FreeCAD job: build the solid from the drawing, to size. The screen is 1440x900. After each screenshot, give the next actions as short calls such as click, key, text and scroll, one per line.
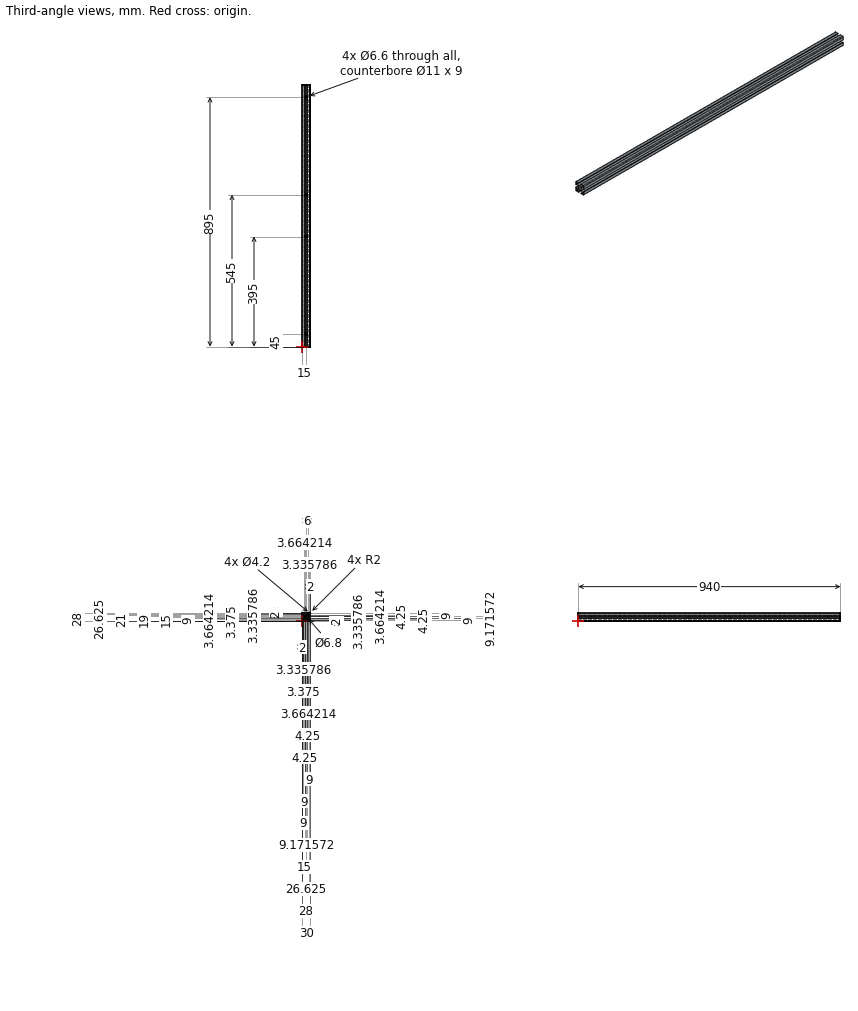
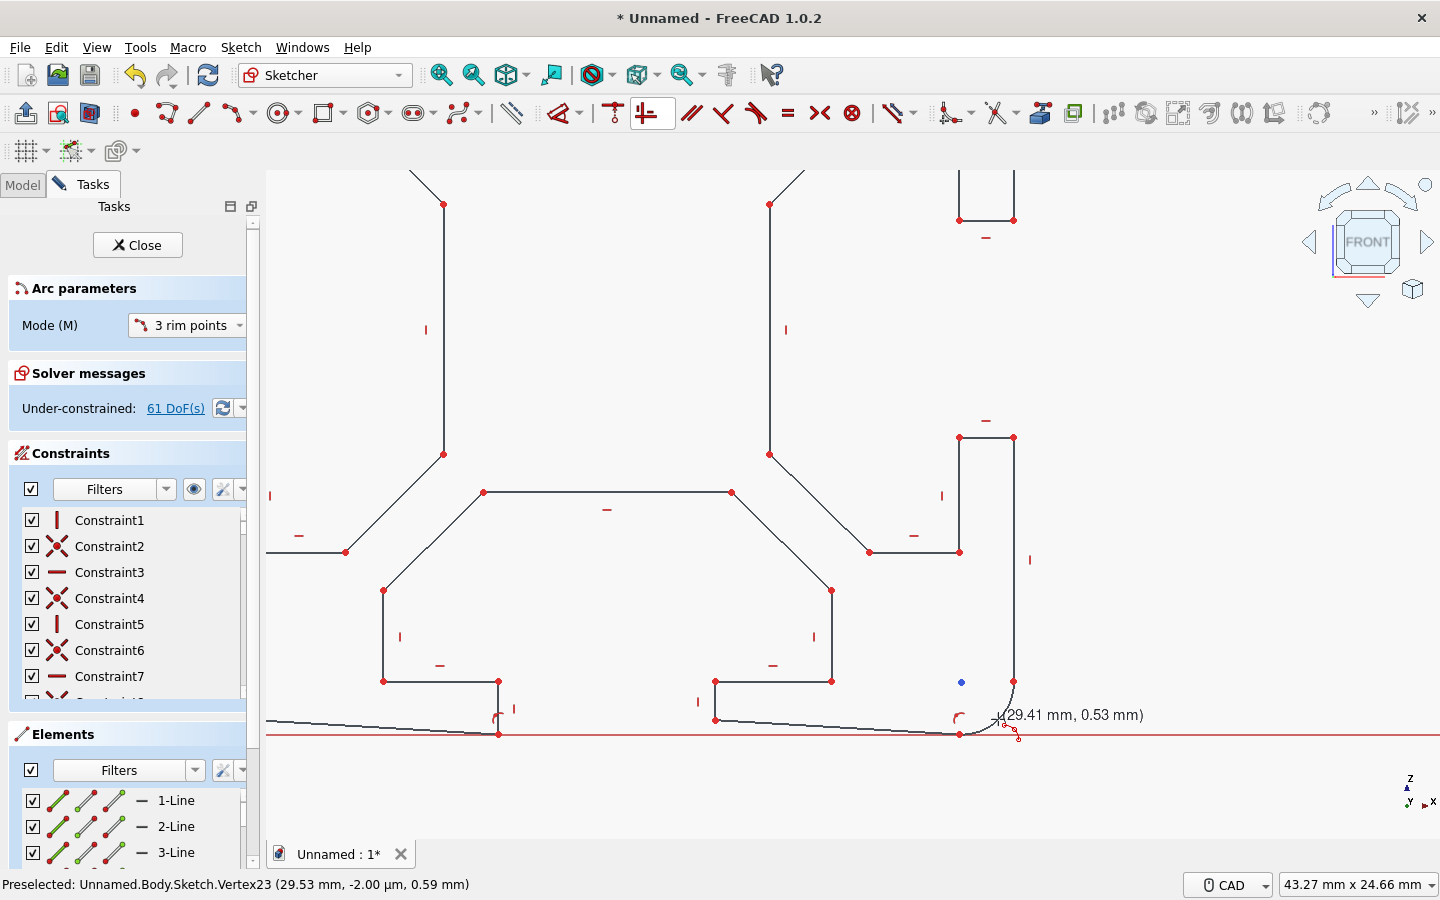
scroll(1000, 720, down, 3)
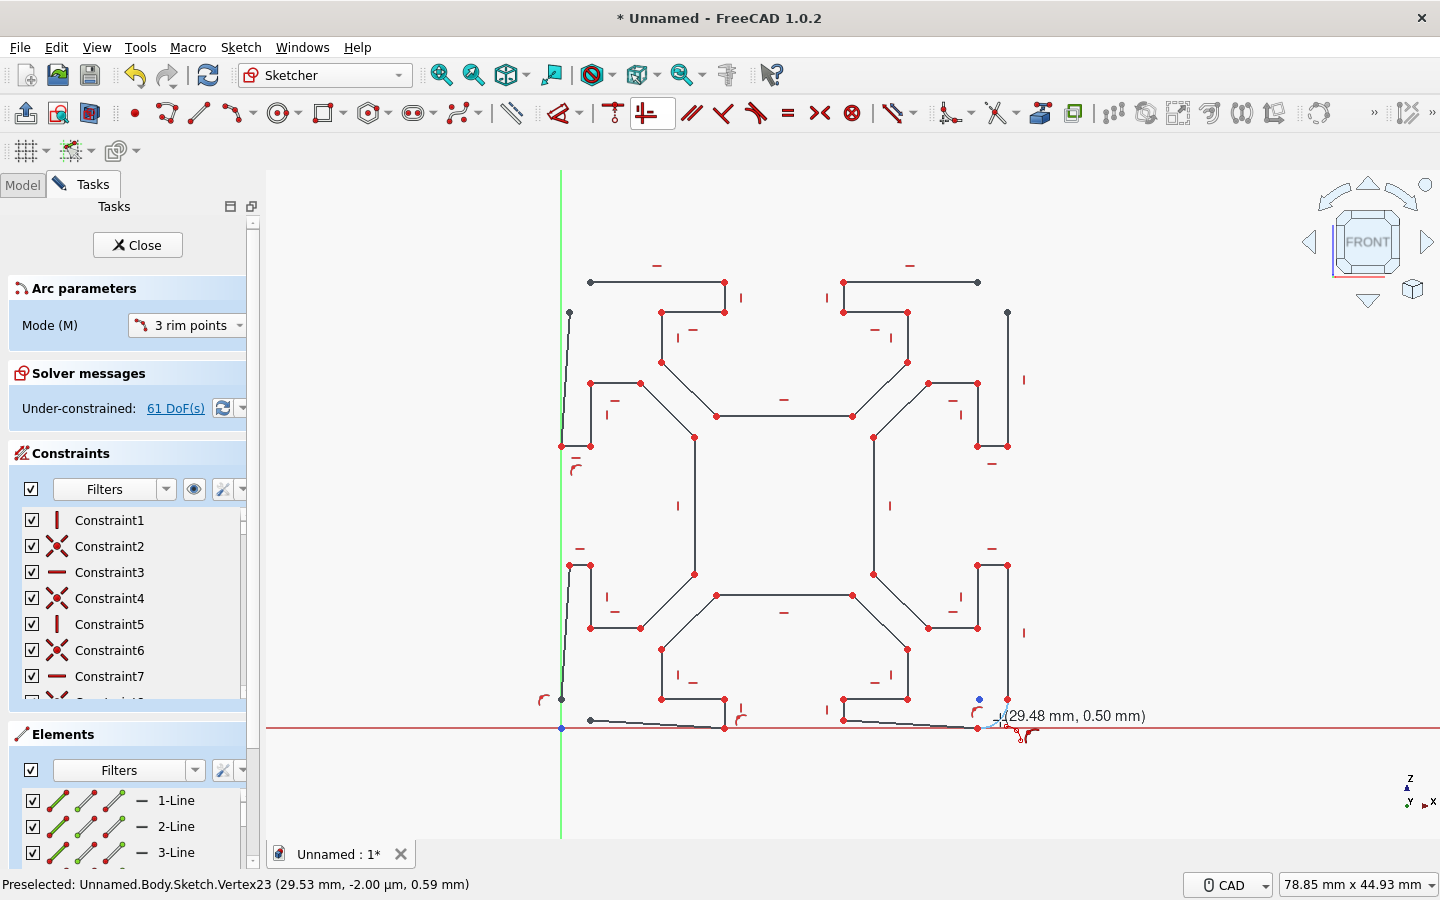
click(591, 720)
click(561, 699)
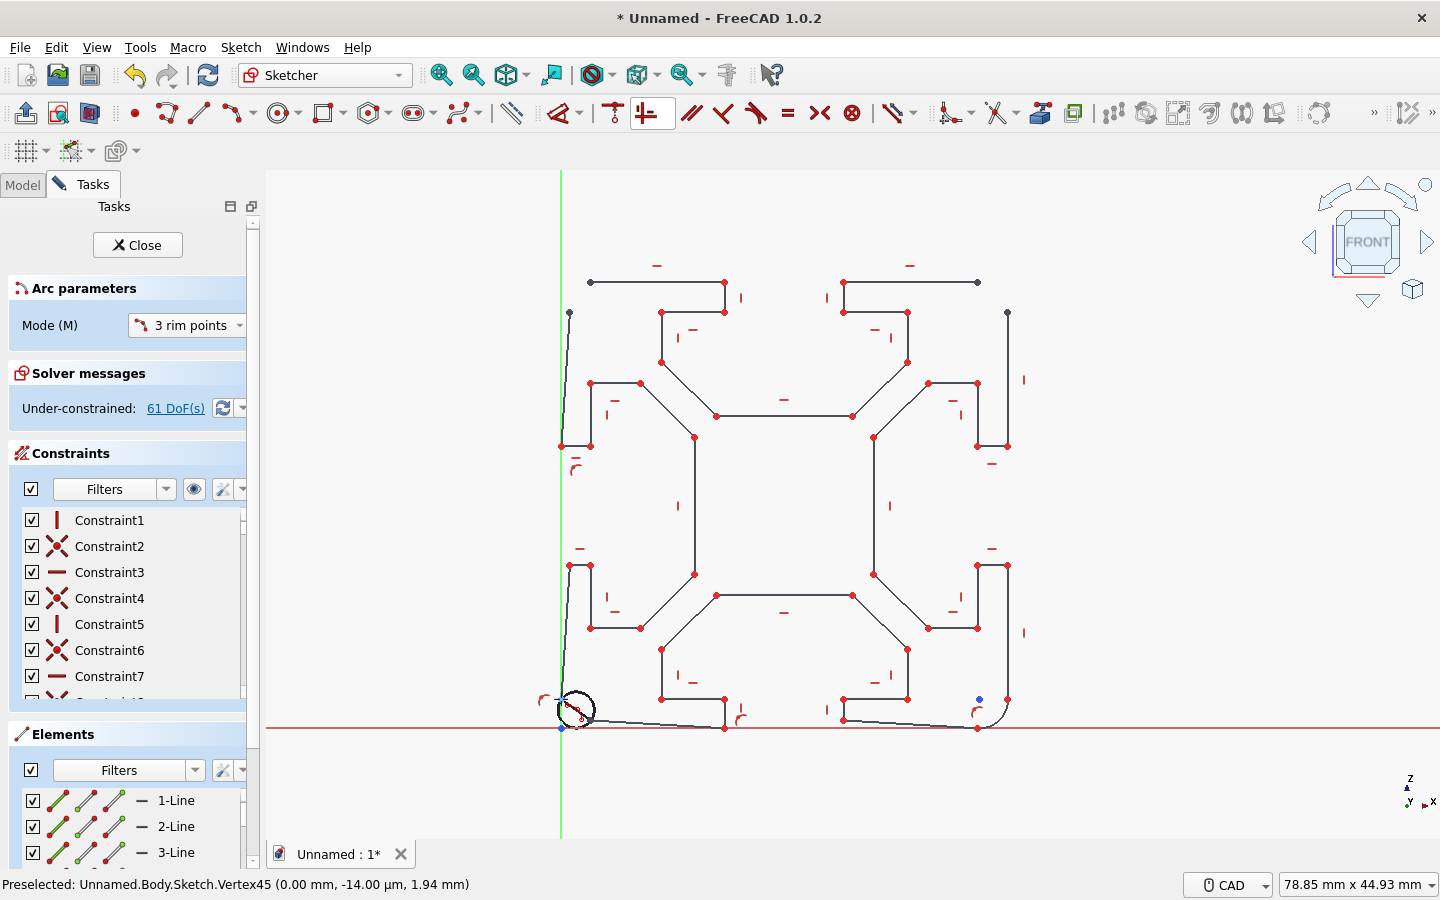
scroll(570, 720, up, 3)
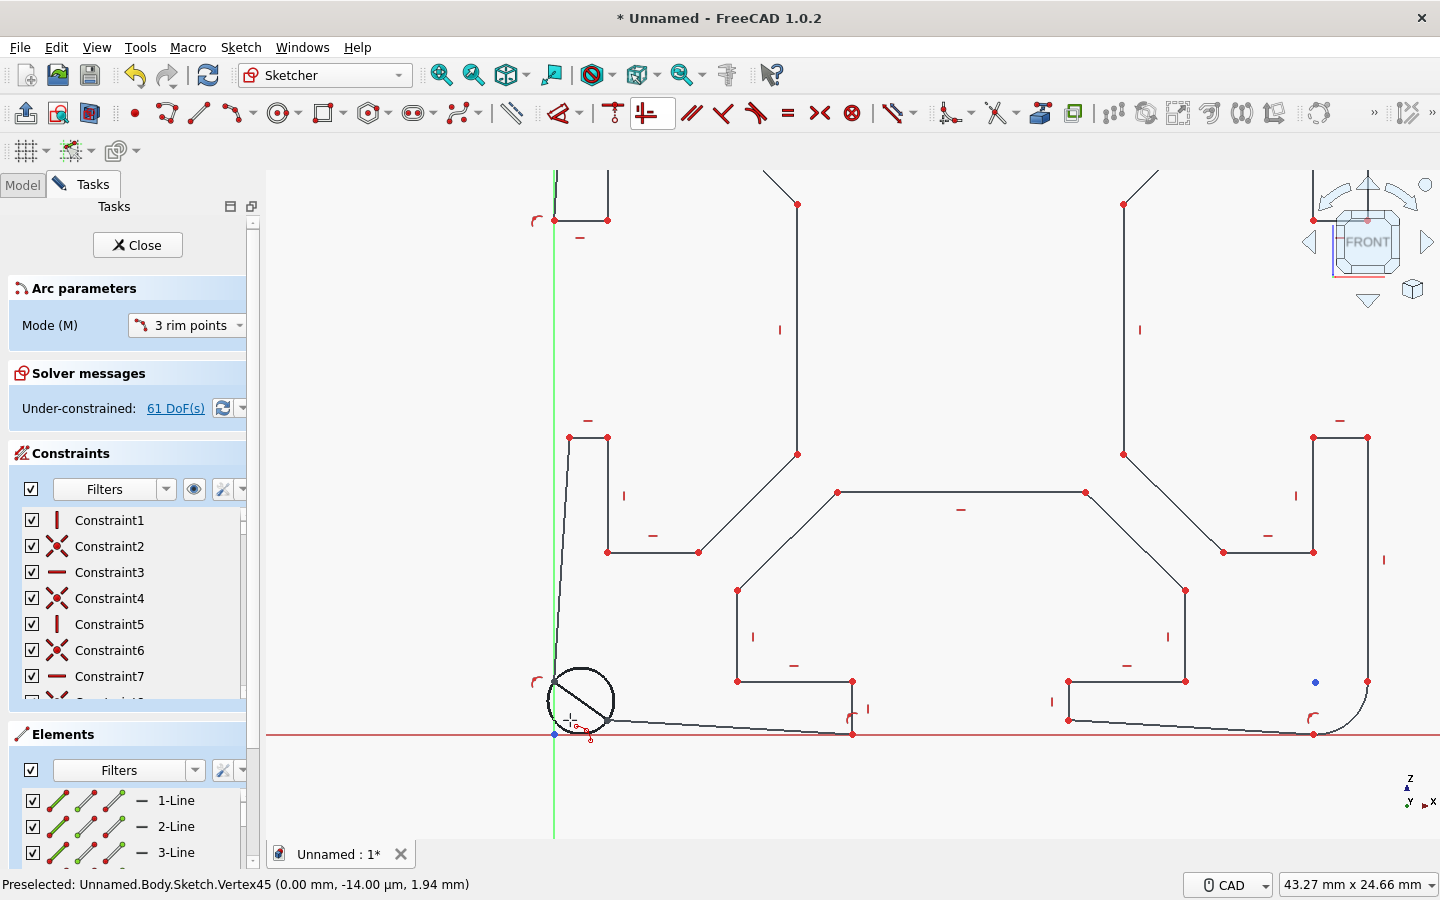
click(570, 719)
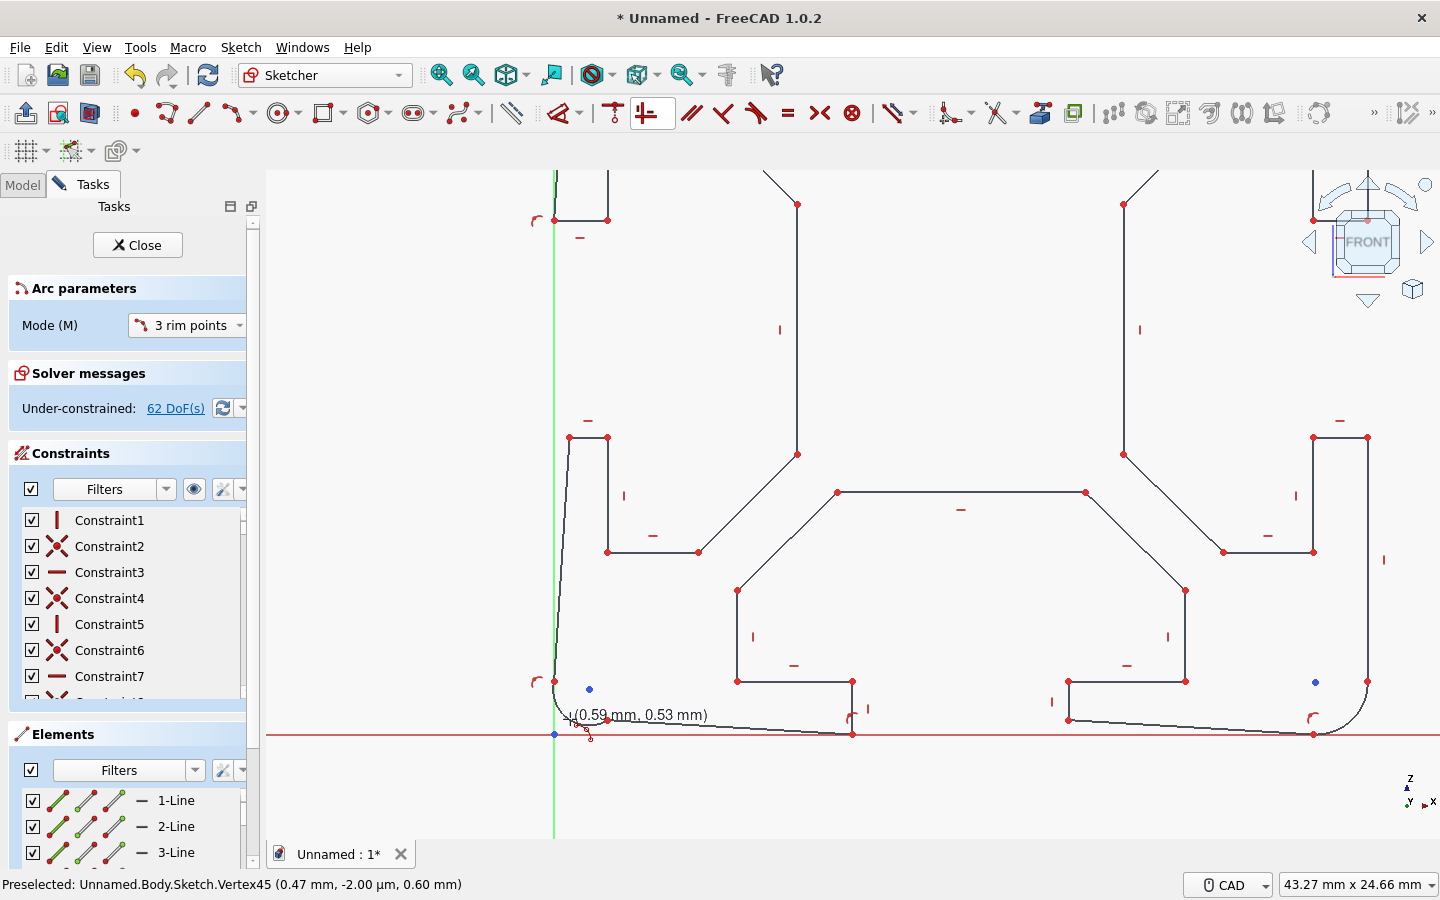
scroll(570, 720, down, 3)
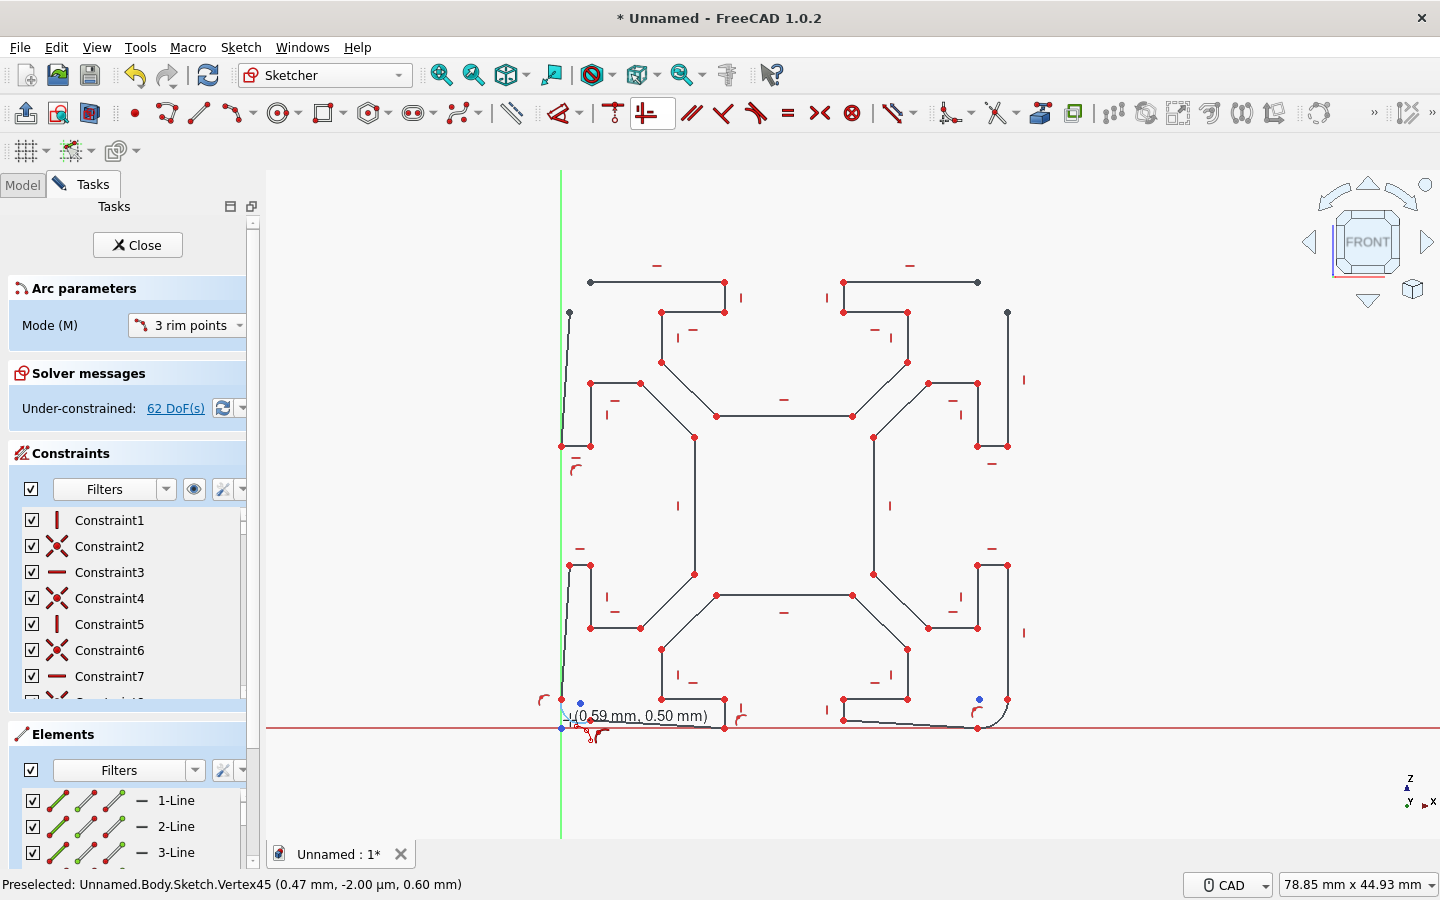
click(570, 312)
click(591, 282)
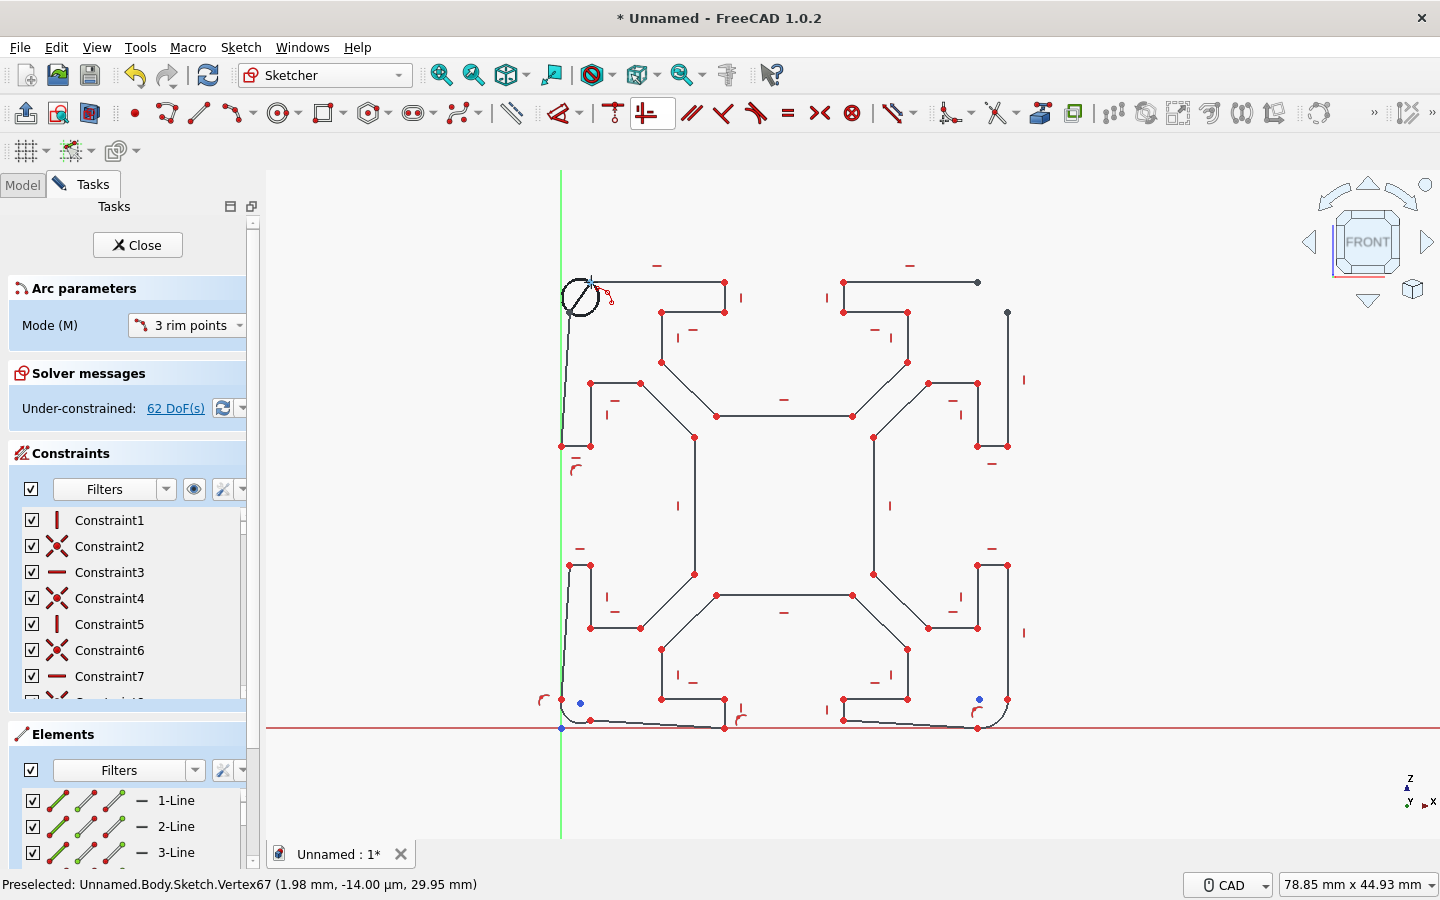
scroll(570, 290, up, 3)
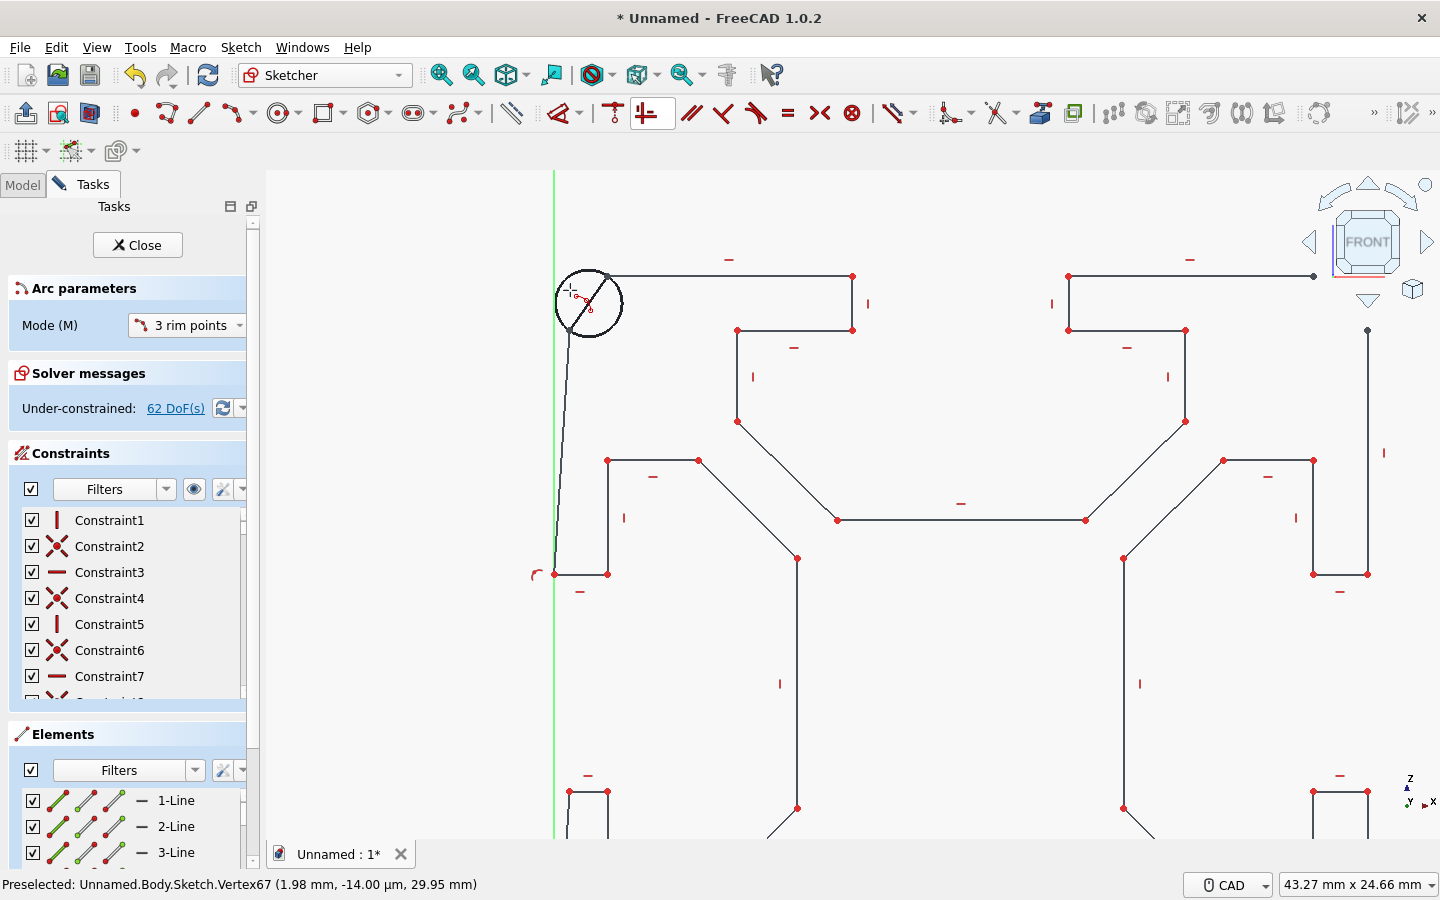
click(570, 291)